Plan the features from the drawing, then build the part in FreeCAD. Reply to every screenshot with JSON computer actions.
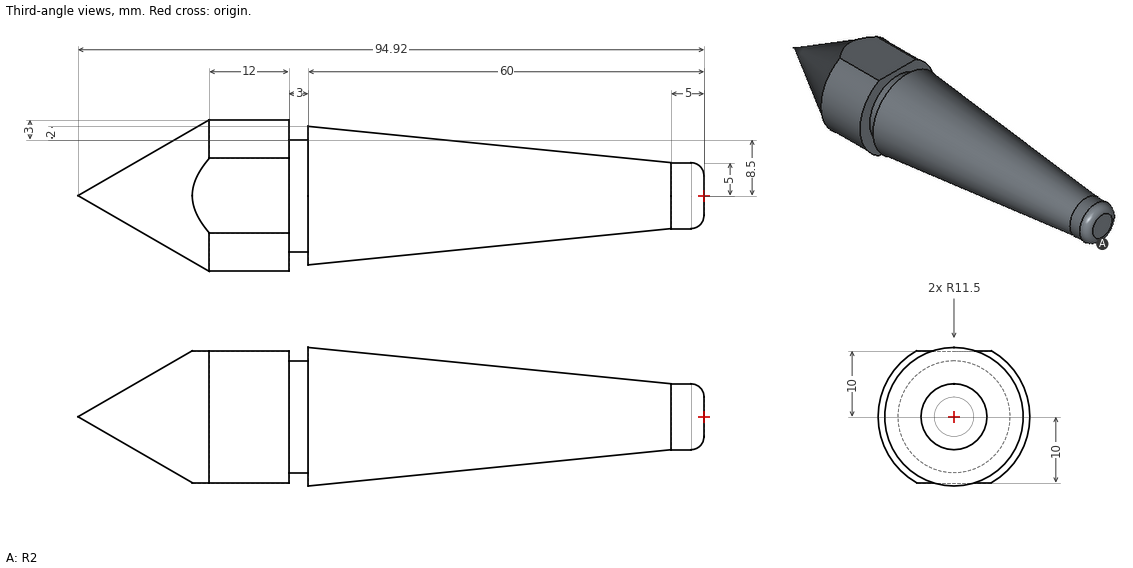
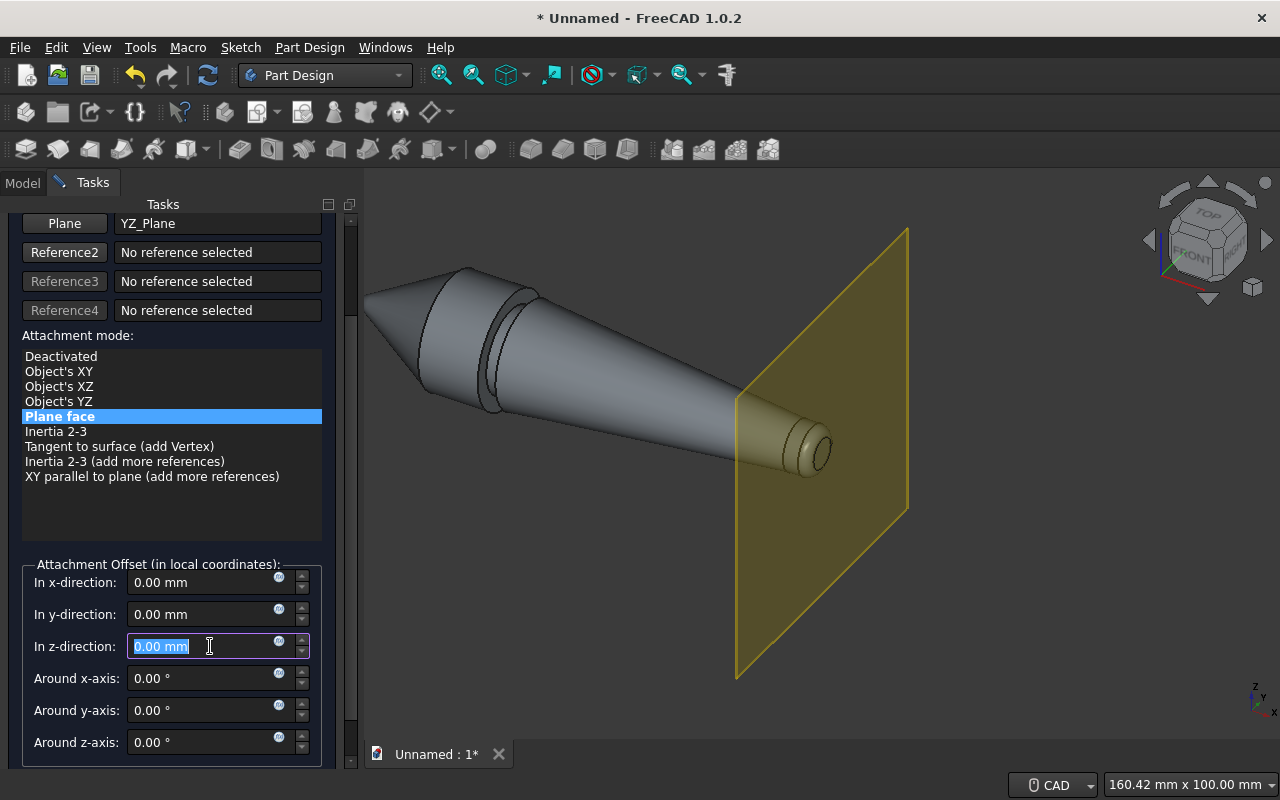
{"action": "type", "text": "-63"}
{"action": "key", "text": "Tab"}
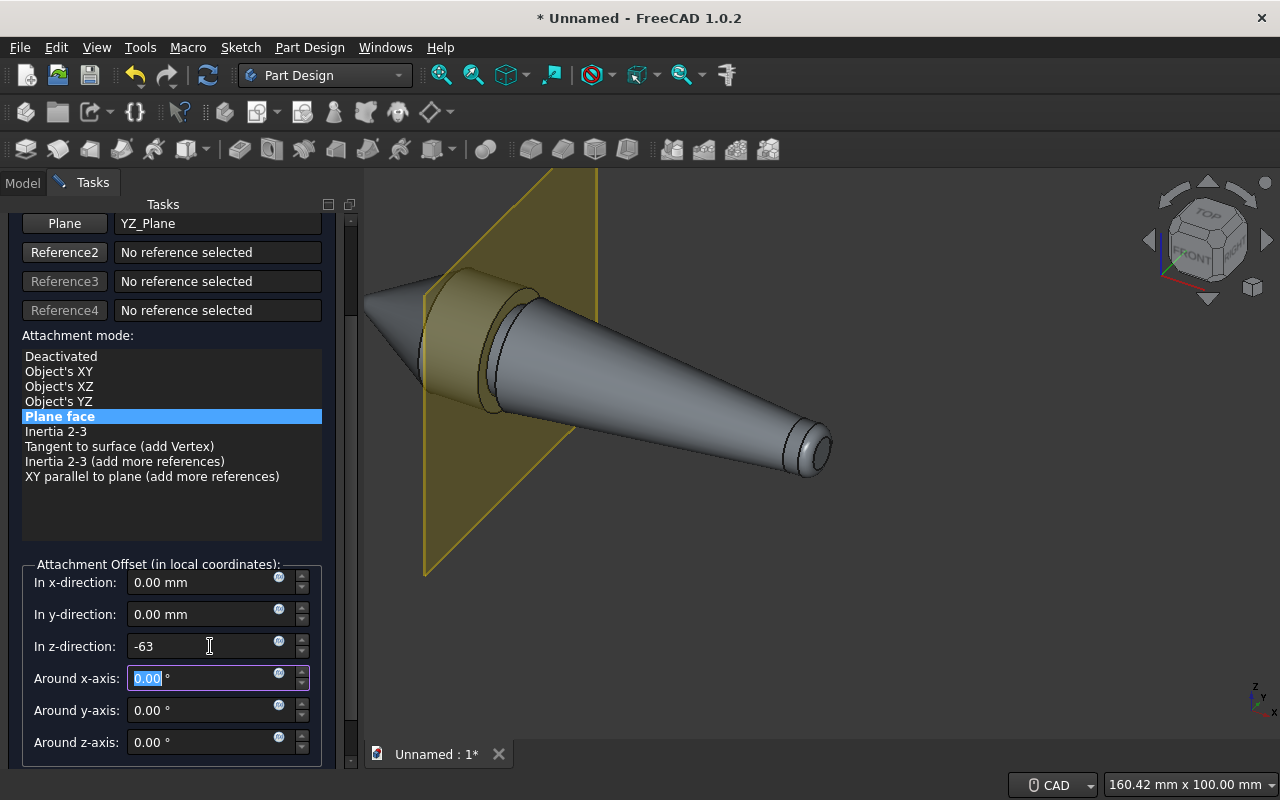
{"action": "scroll", "coordinate": [351, 491], "scroll_direction": "up", "scroll_amount": 3}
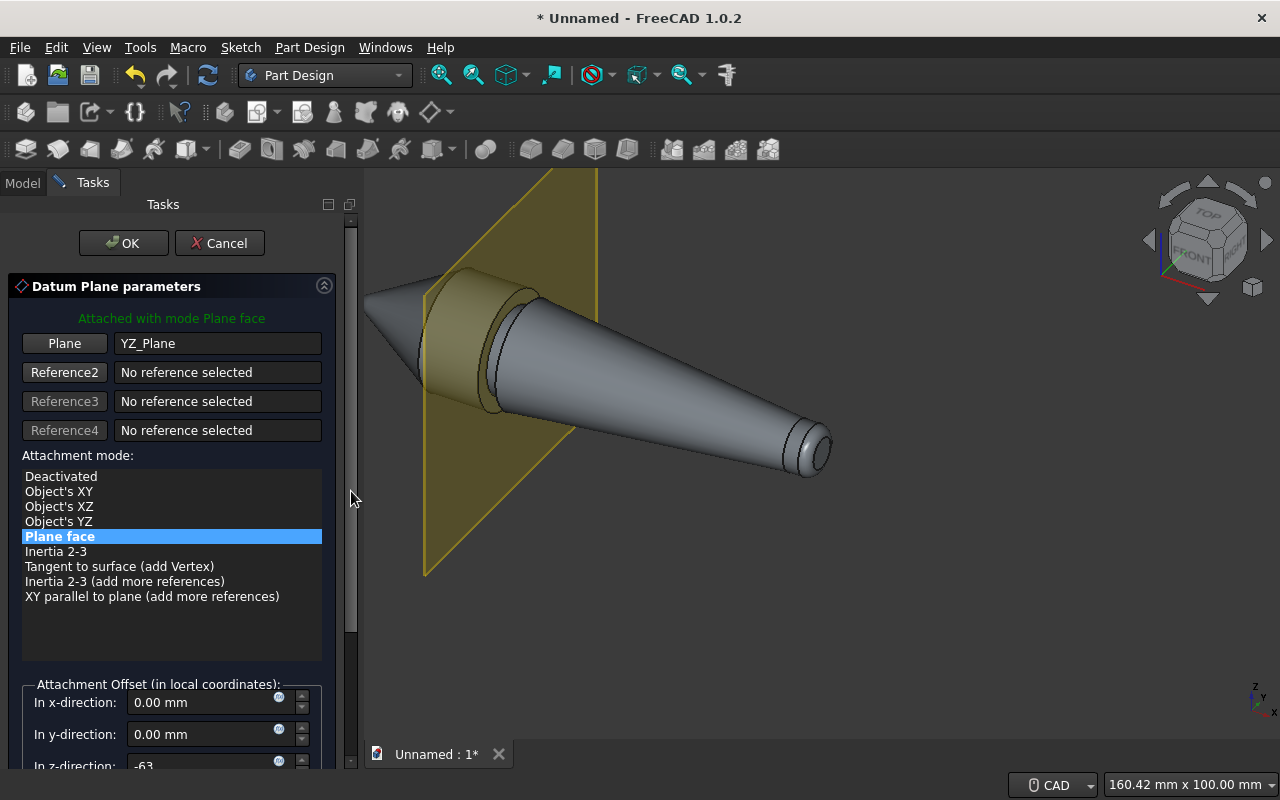
{"action": "left_click", "coordinate": [124, 243]}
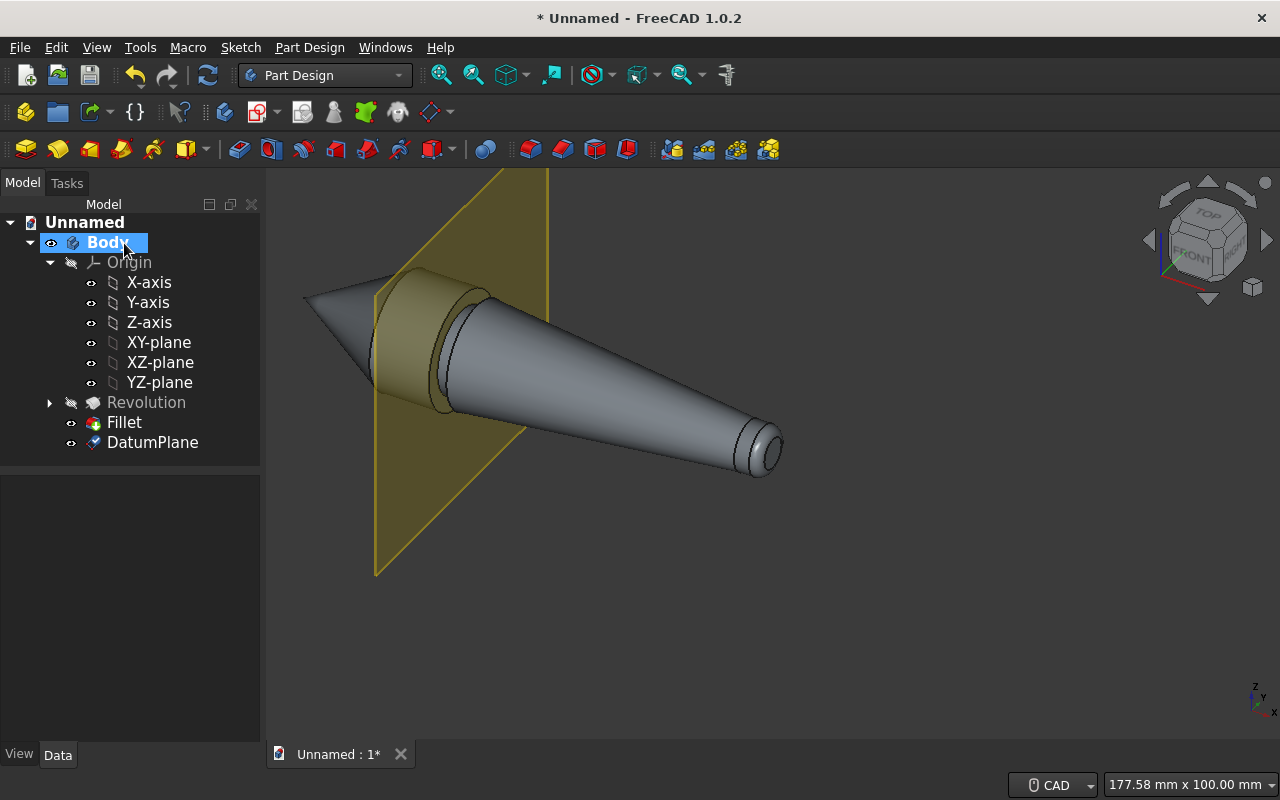
{"action": "left_click", "coordinate": [116, 443]}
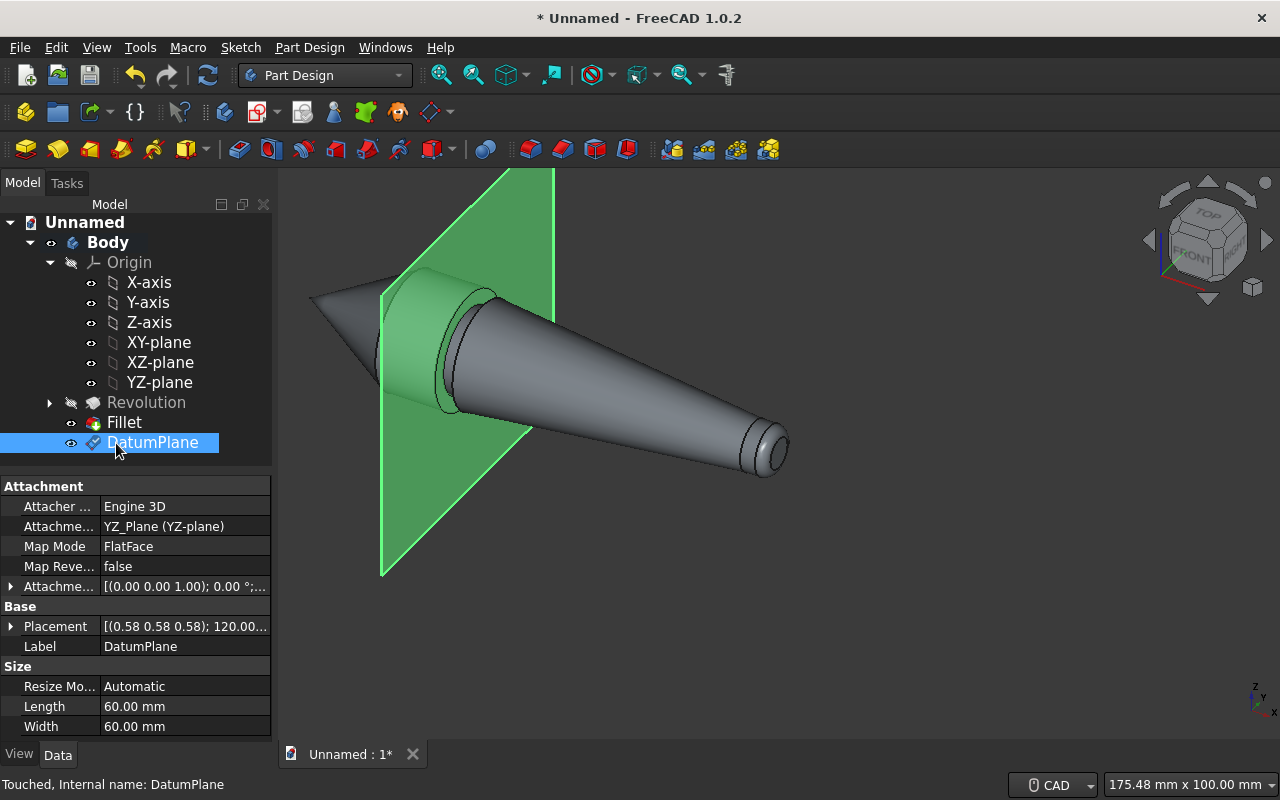
{"action": "left_click", "coordinate": [258, 112]}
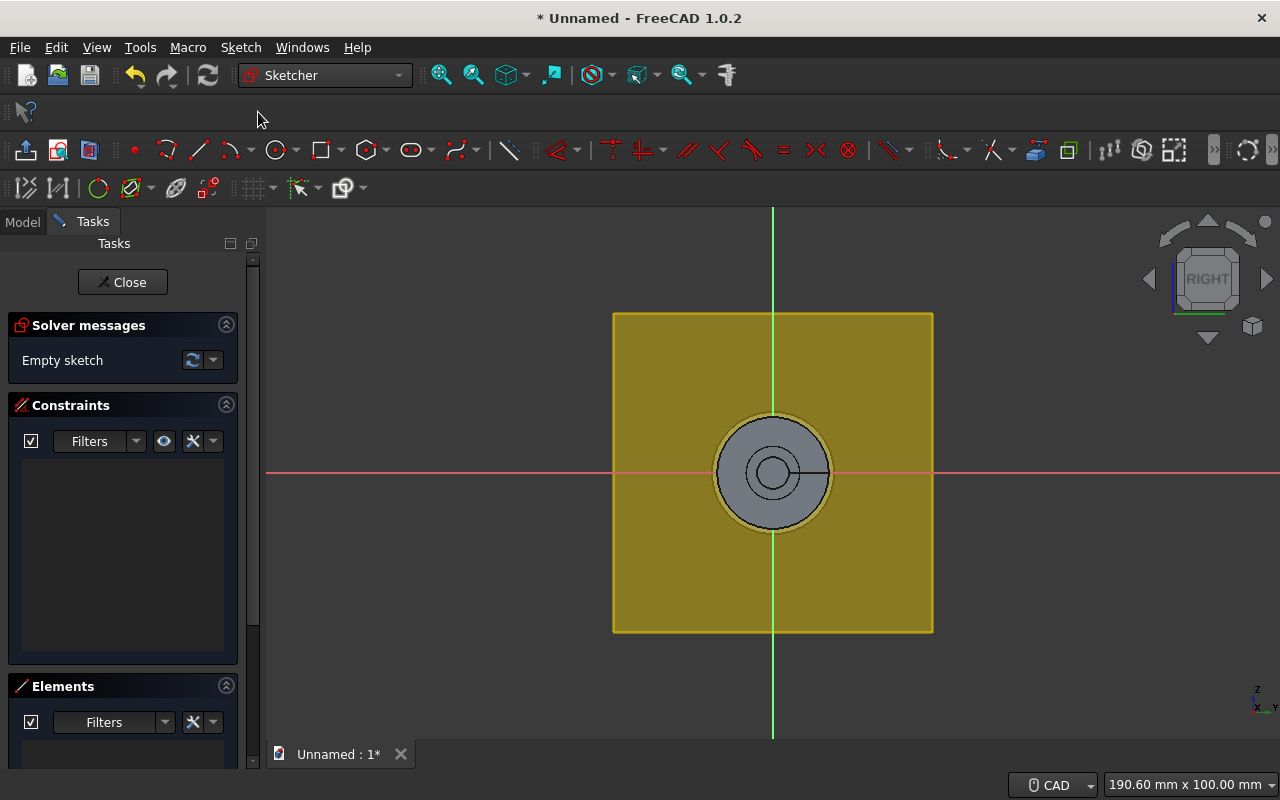
{"action": "left_click", "coordinate": [90, 150]}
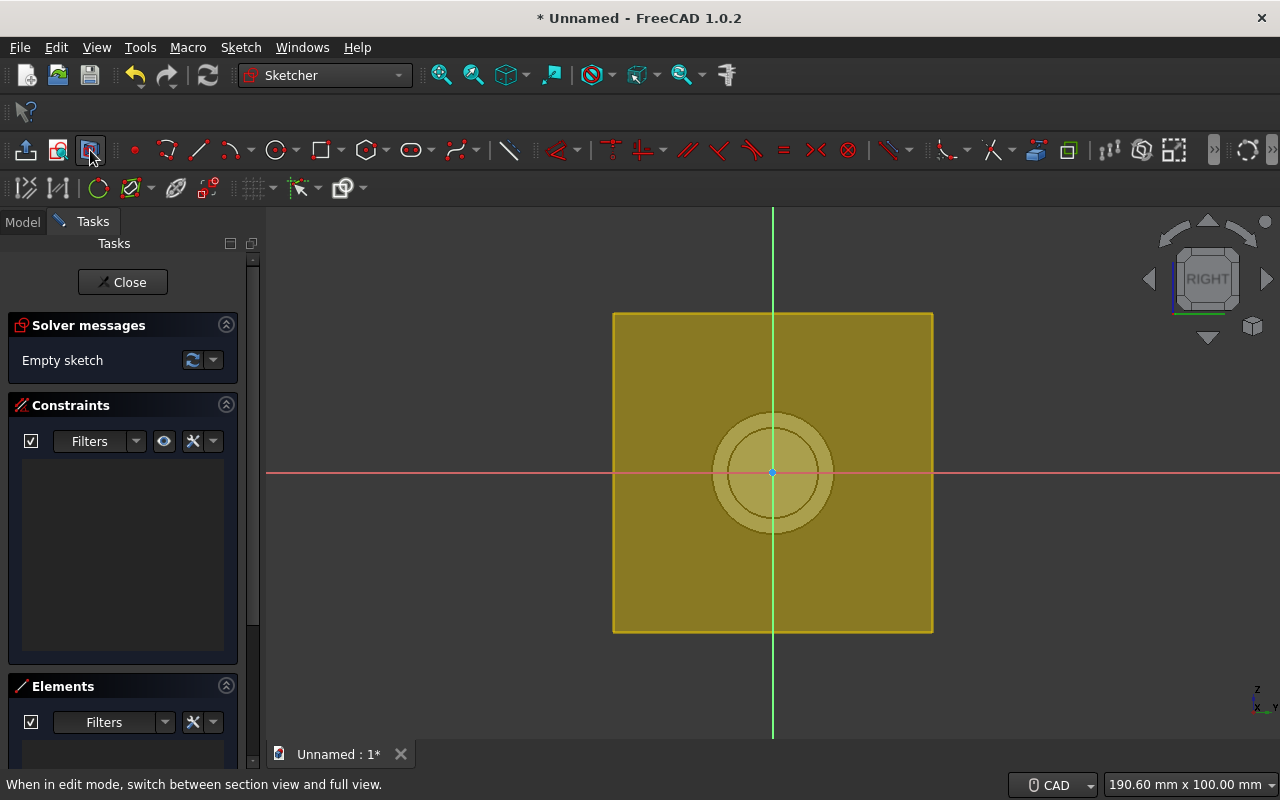
{"action": "scroll", "coordinate": [813, 473], "scroll_direction": "up", "scroll_amount": 5}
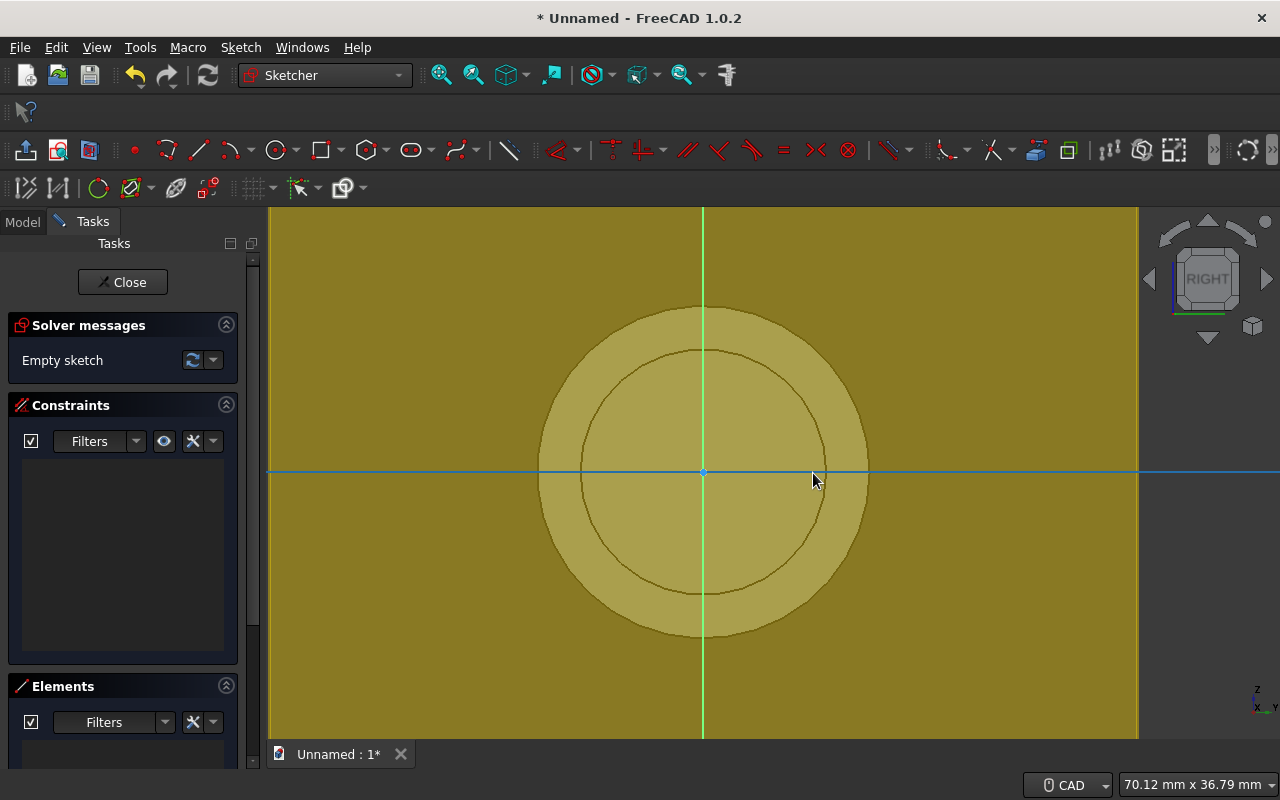
{"action": "left_click", "coordinate": [200, 150]}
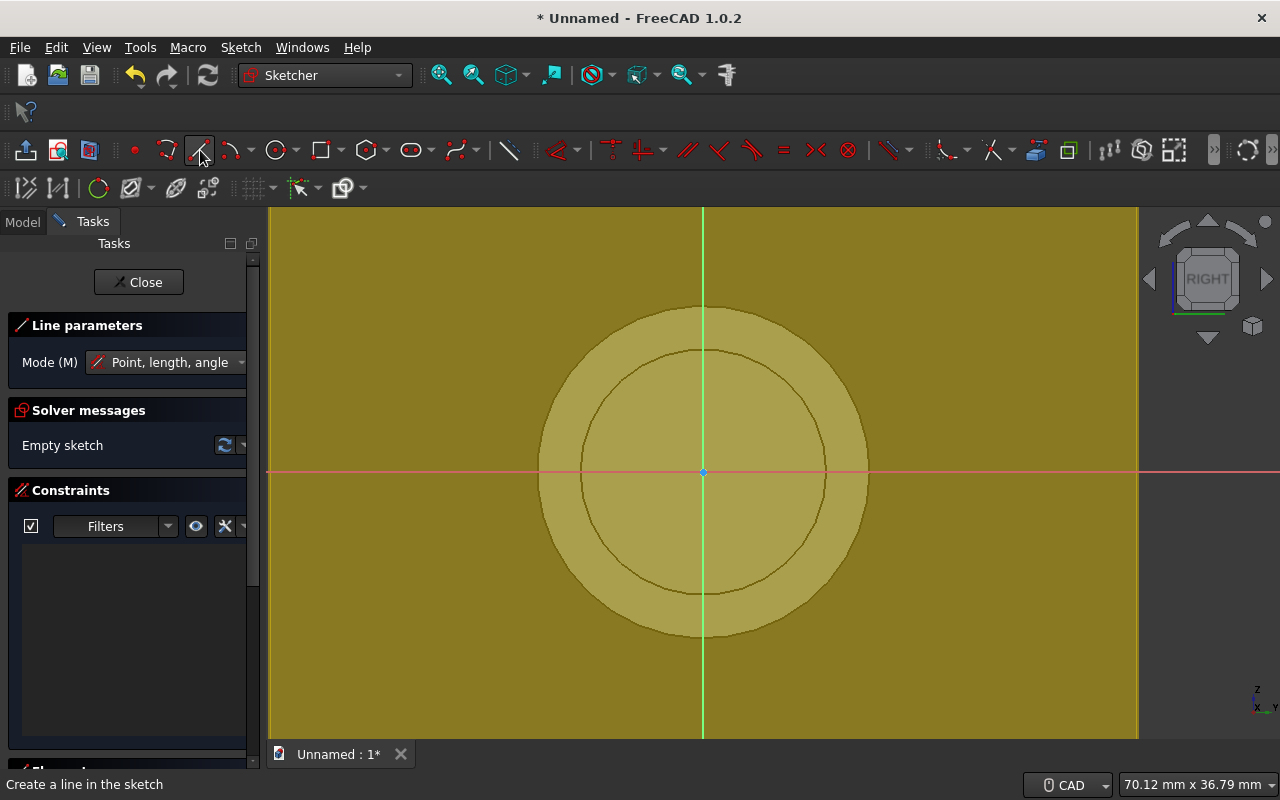
{"action": "left_click", "coordinate": [621, 328]}
{"action": "left_click", "coordinate": [785, 328]}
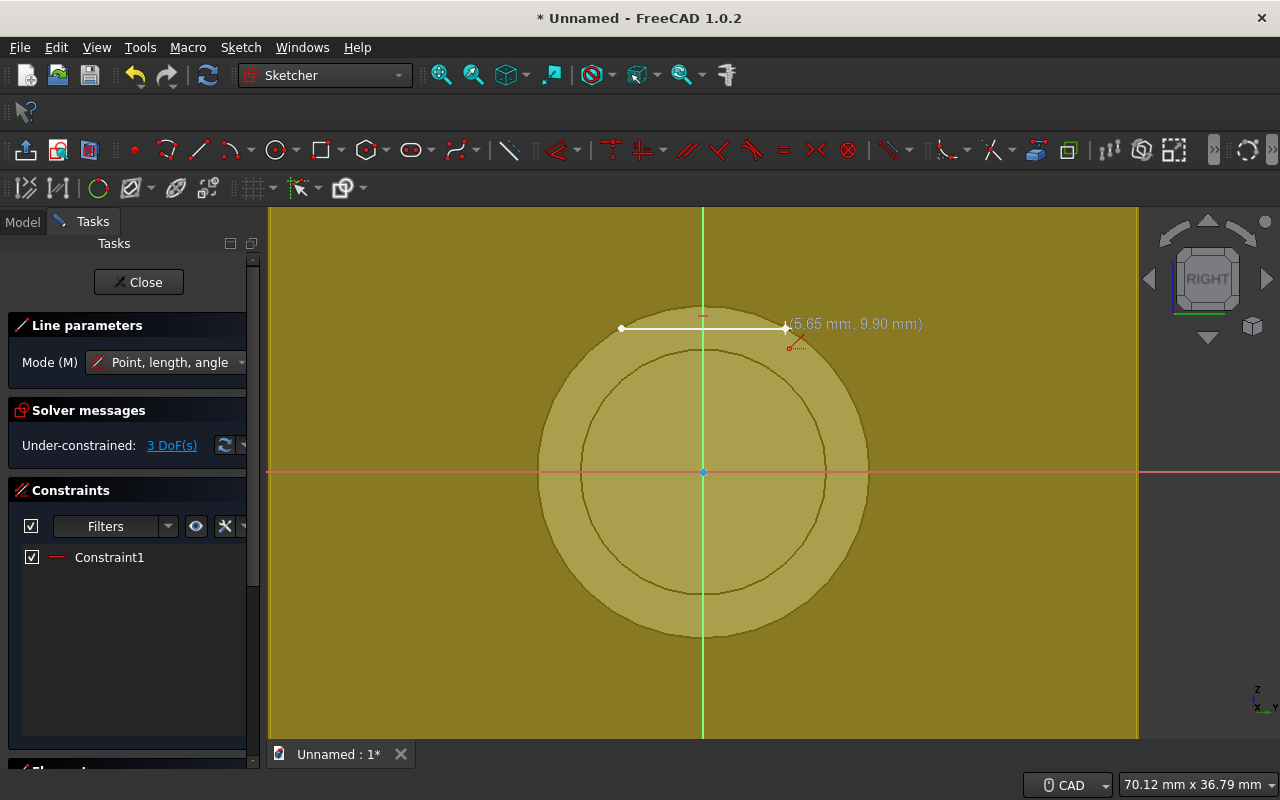
{"action": "left_click", "coordinate": [254, 150]}